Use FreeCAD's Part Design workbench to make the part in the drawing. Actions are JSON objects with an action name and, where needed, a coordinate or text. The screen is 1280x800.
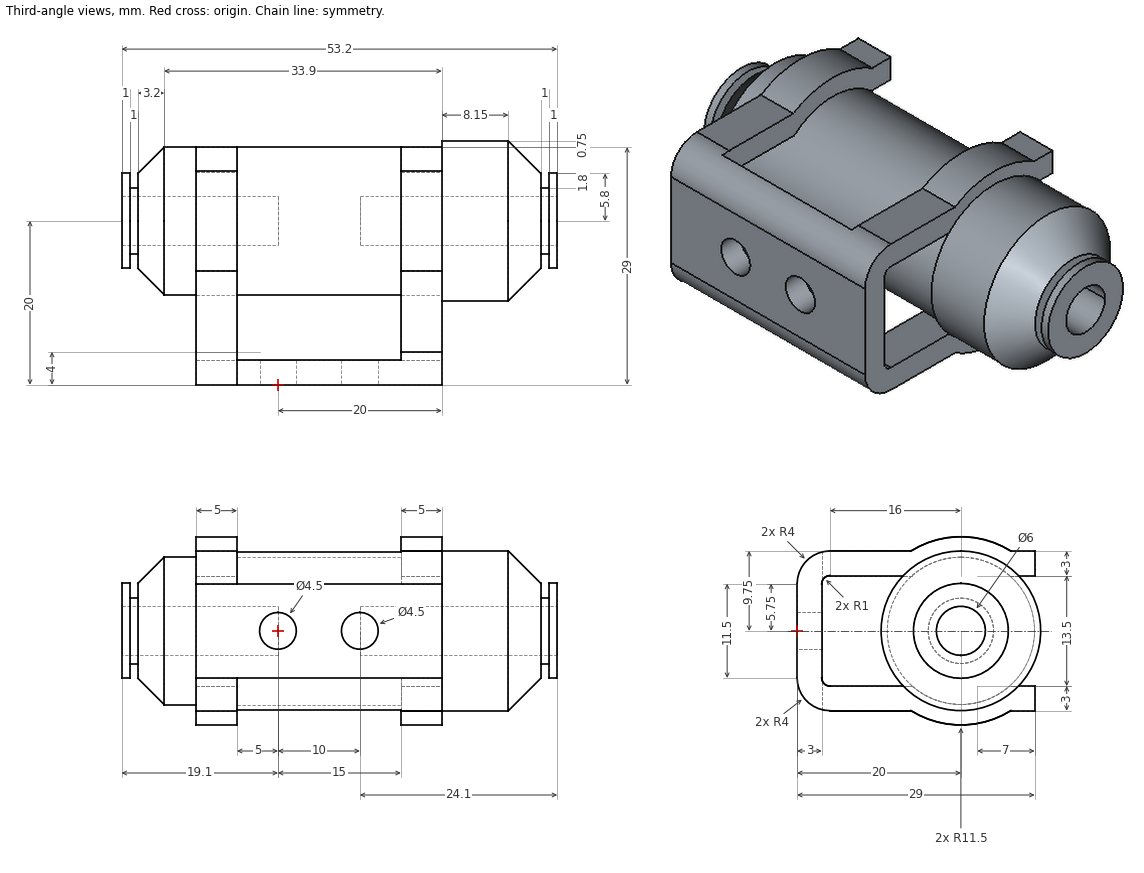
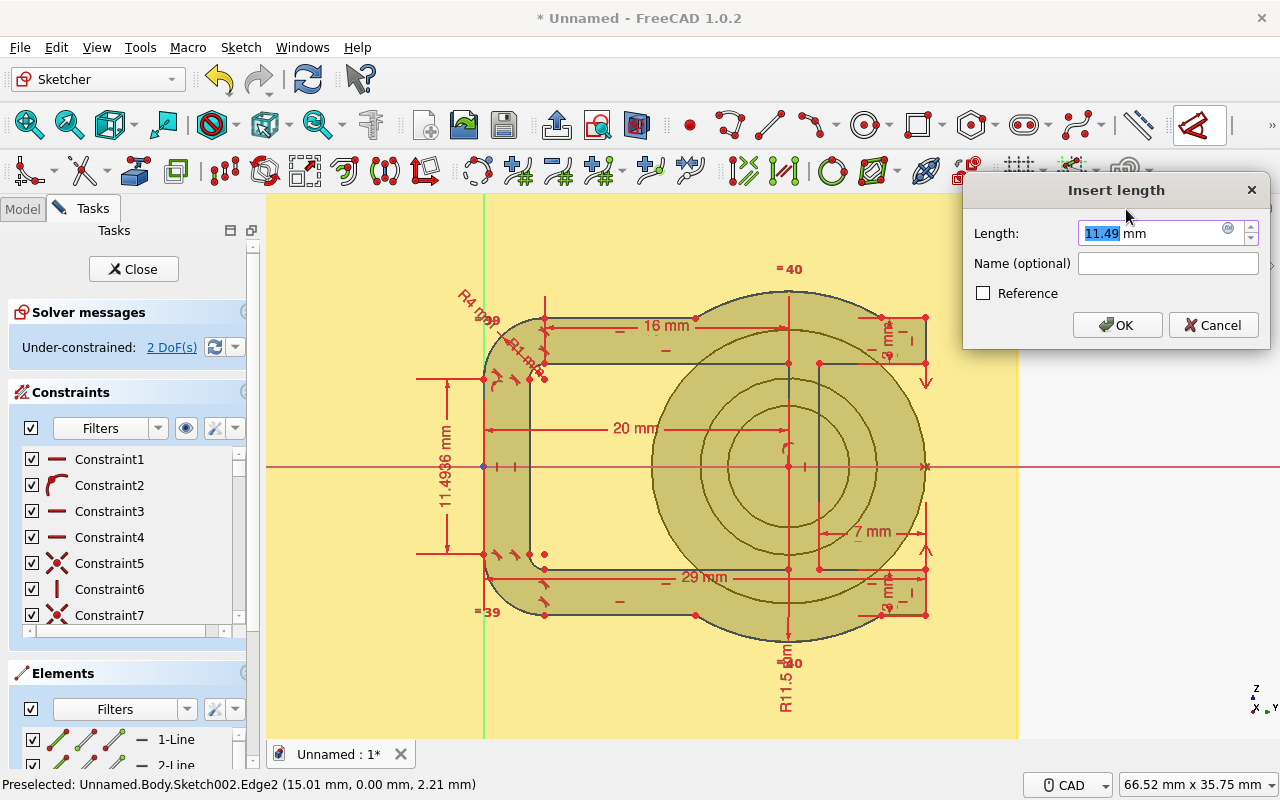
{"action": "type", "text": "11.5"}
{"action": "key", "text": "Return"}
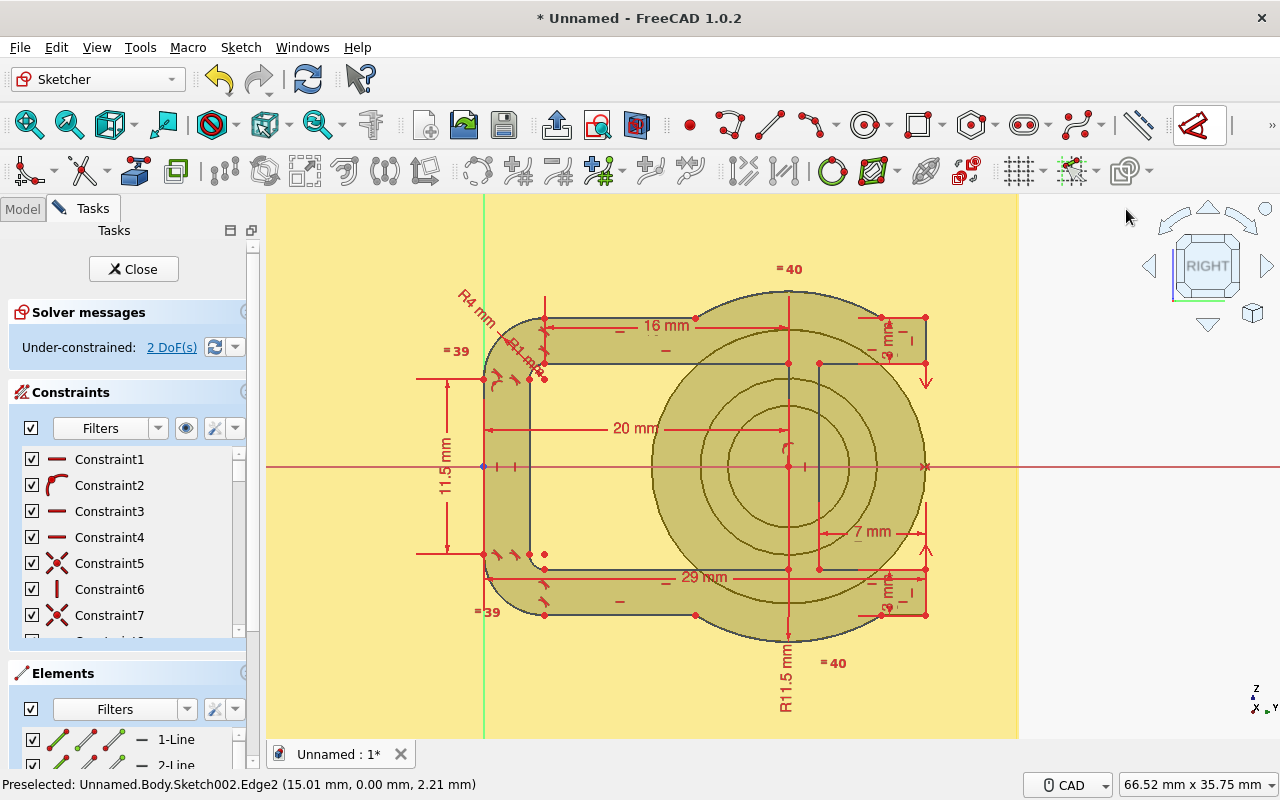
{"action": "left_click", "coordinate": [819, 508]}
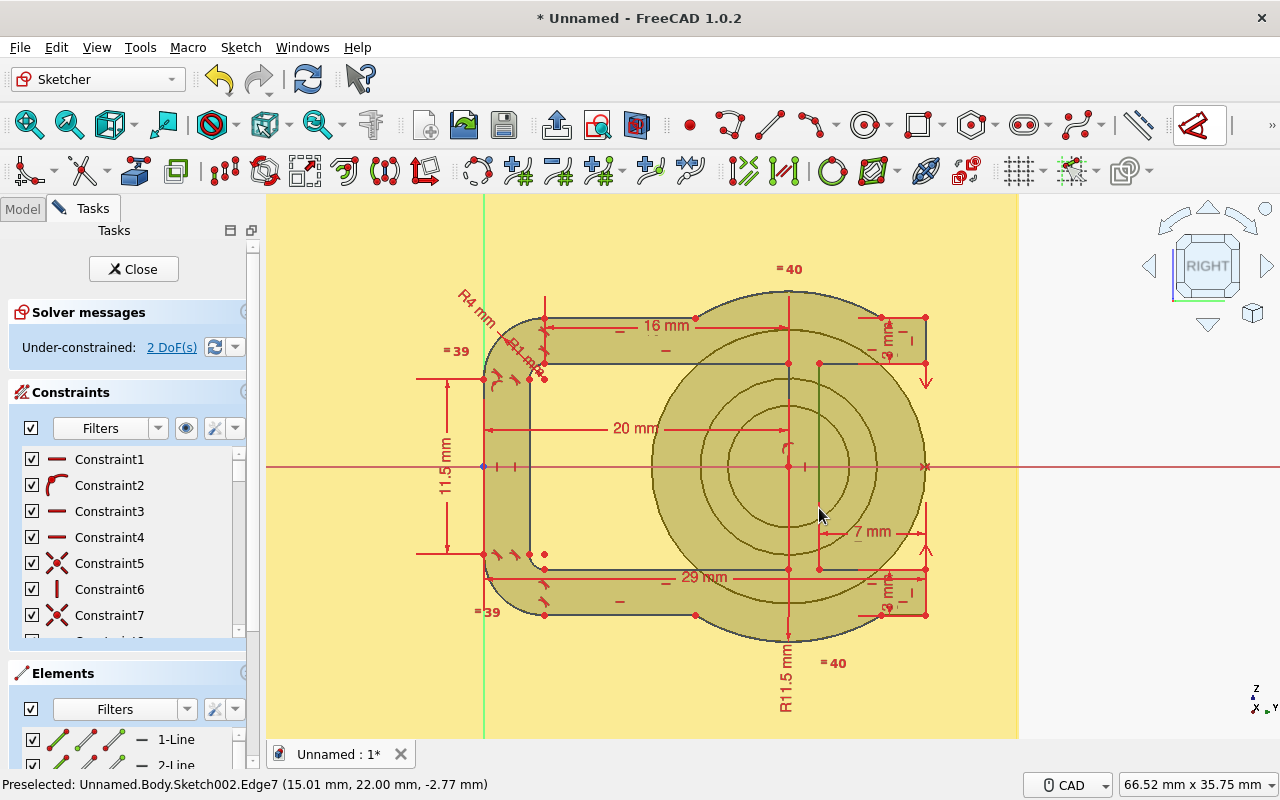
{"action": "left_click", "coordinate": [1220, 126]}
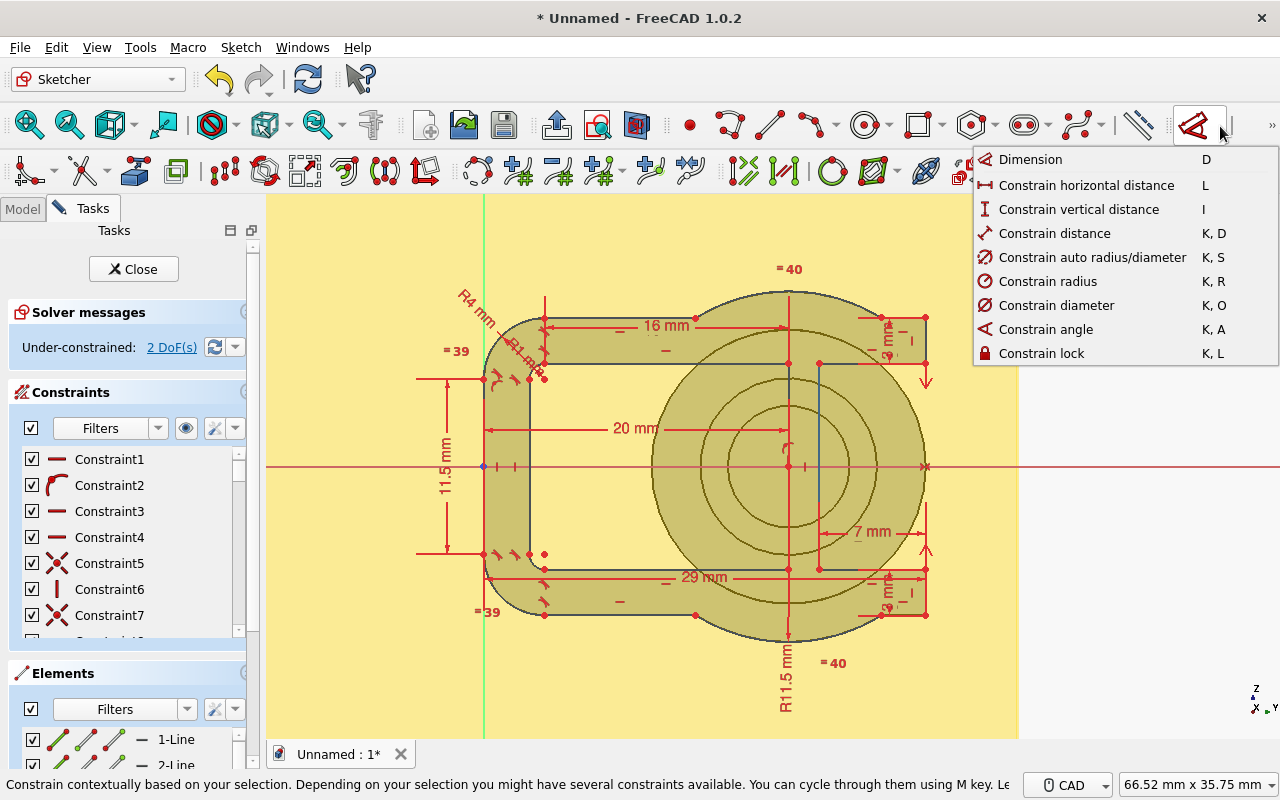
{"action": "left_click", "coordinate": [1126, 209]}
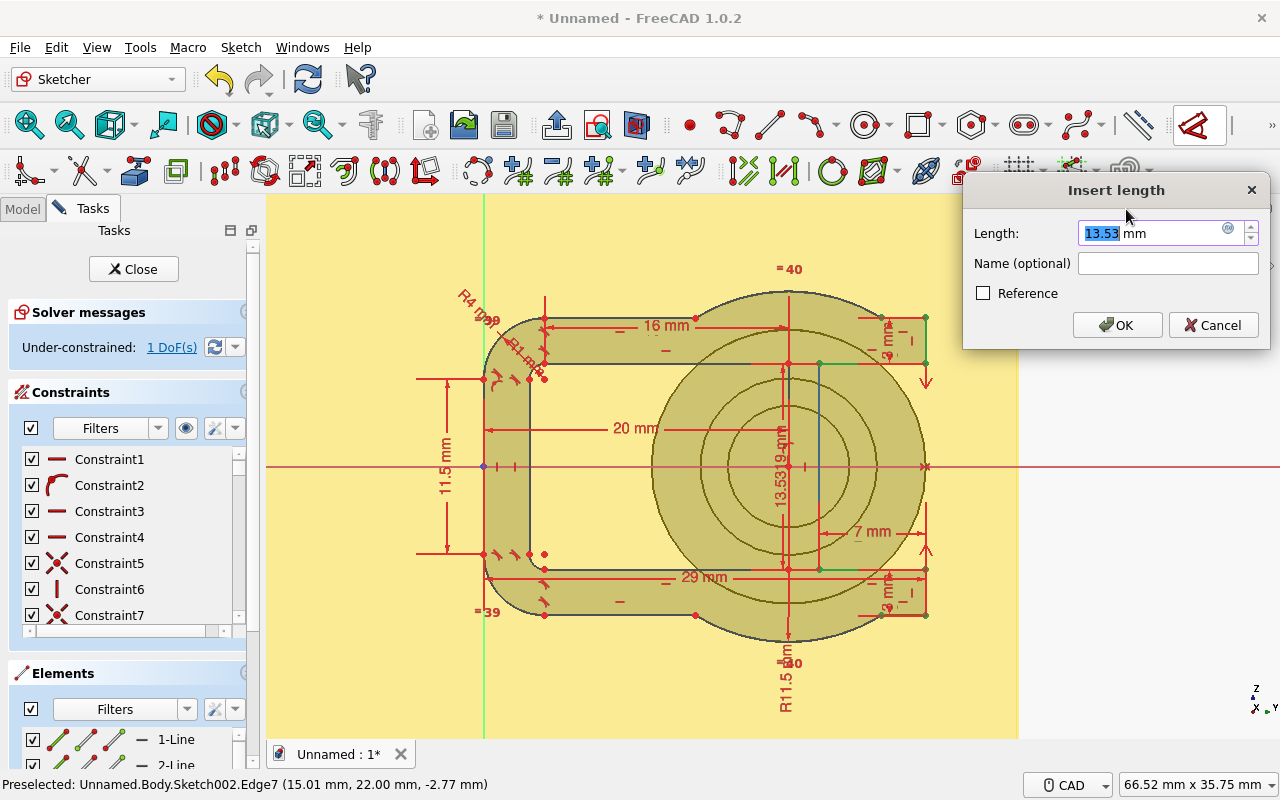
{"action": "type", "text": "13.5"}
{"action": "key", "text": "Return"}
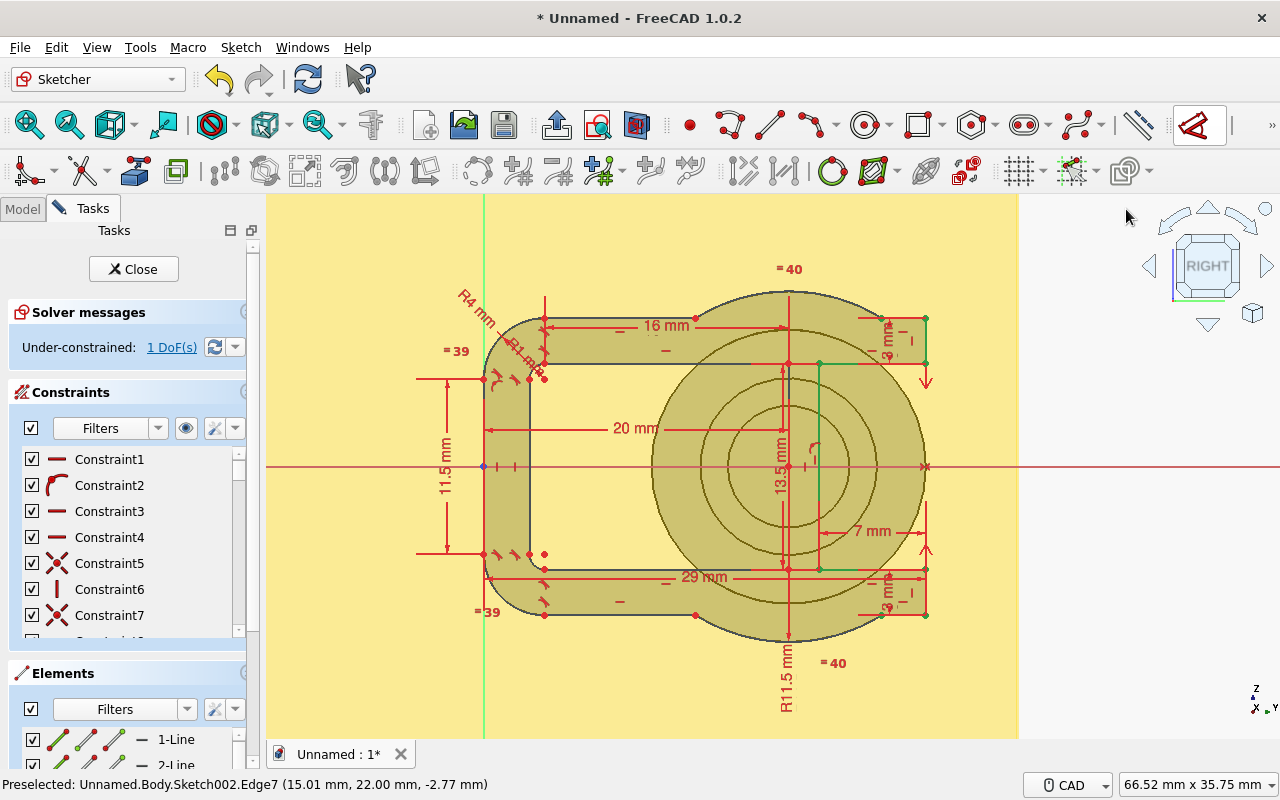
{"action": "left_click", "coordinate": [696, 318]}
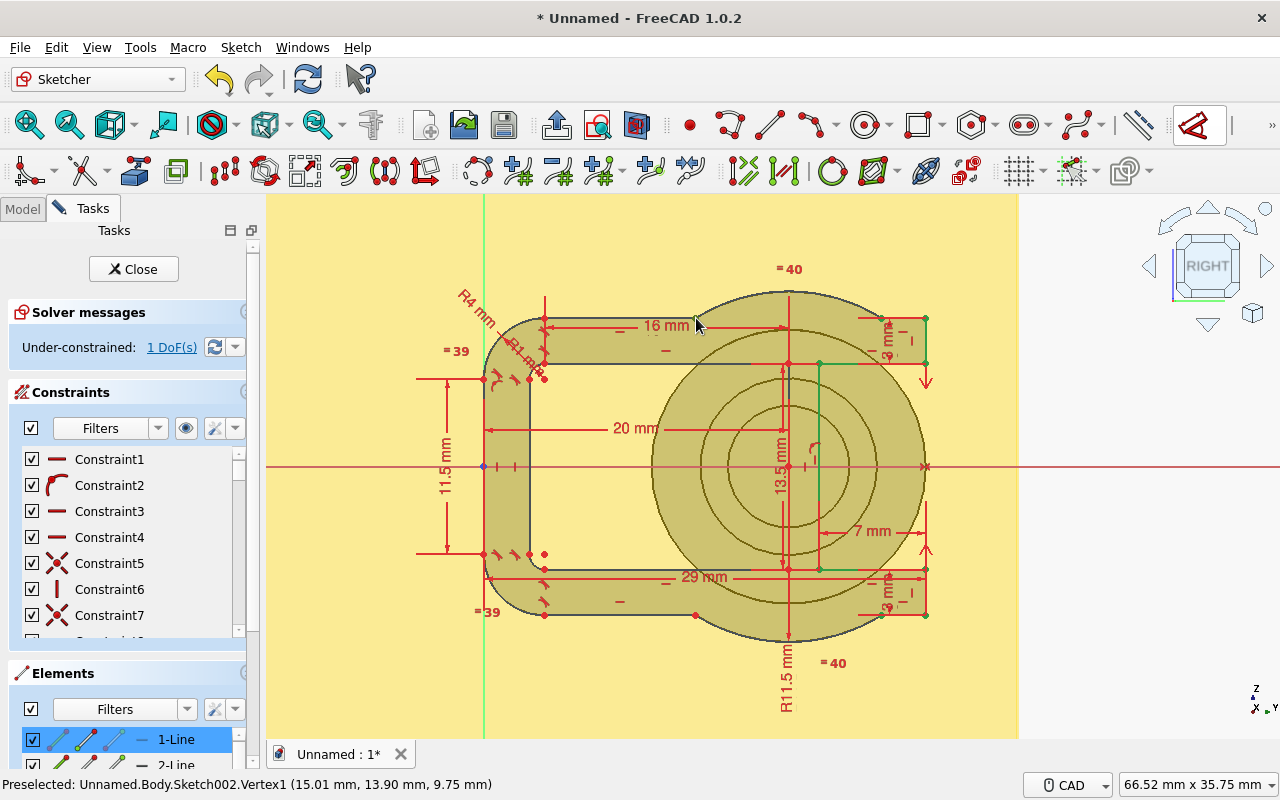
{"action": "left_click", "coordinate": [1220, 126]}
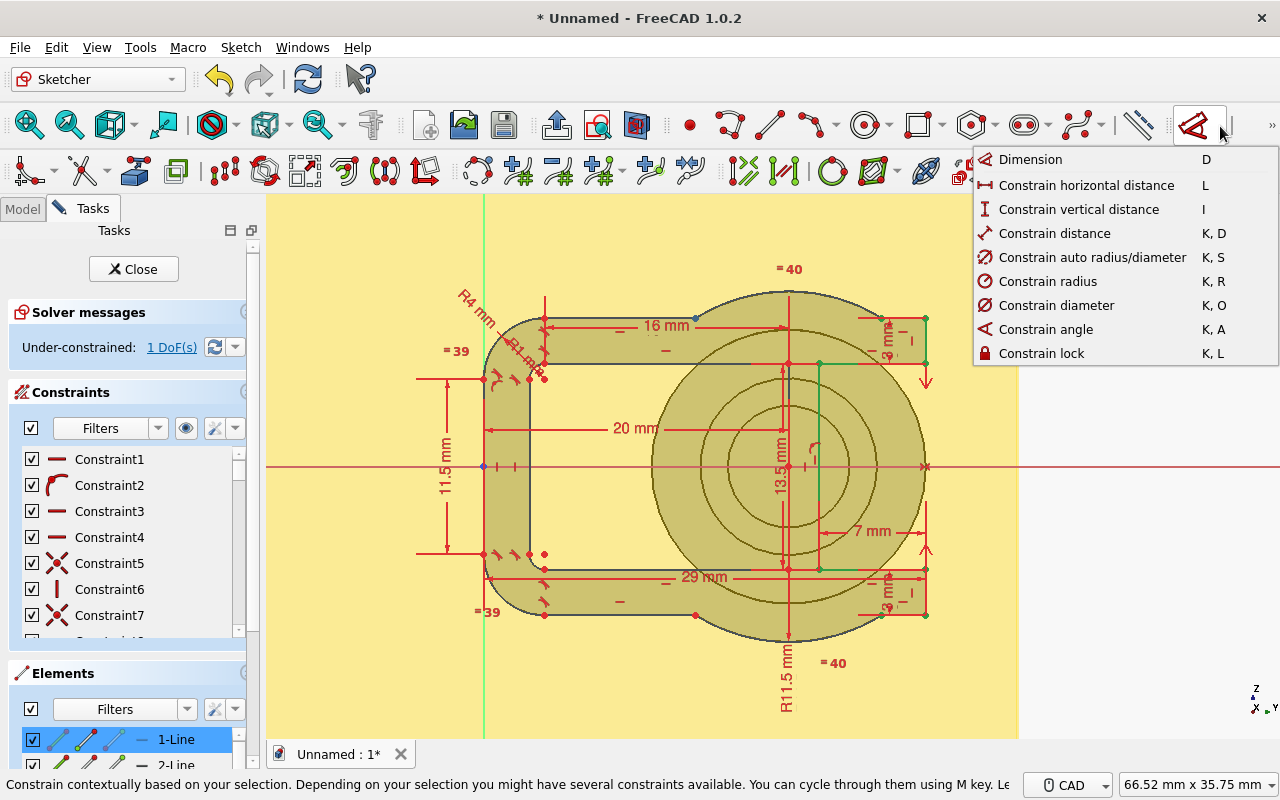
{"action": "left_click", "coordinate": [1126, 209]}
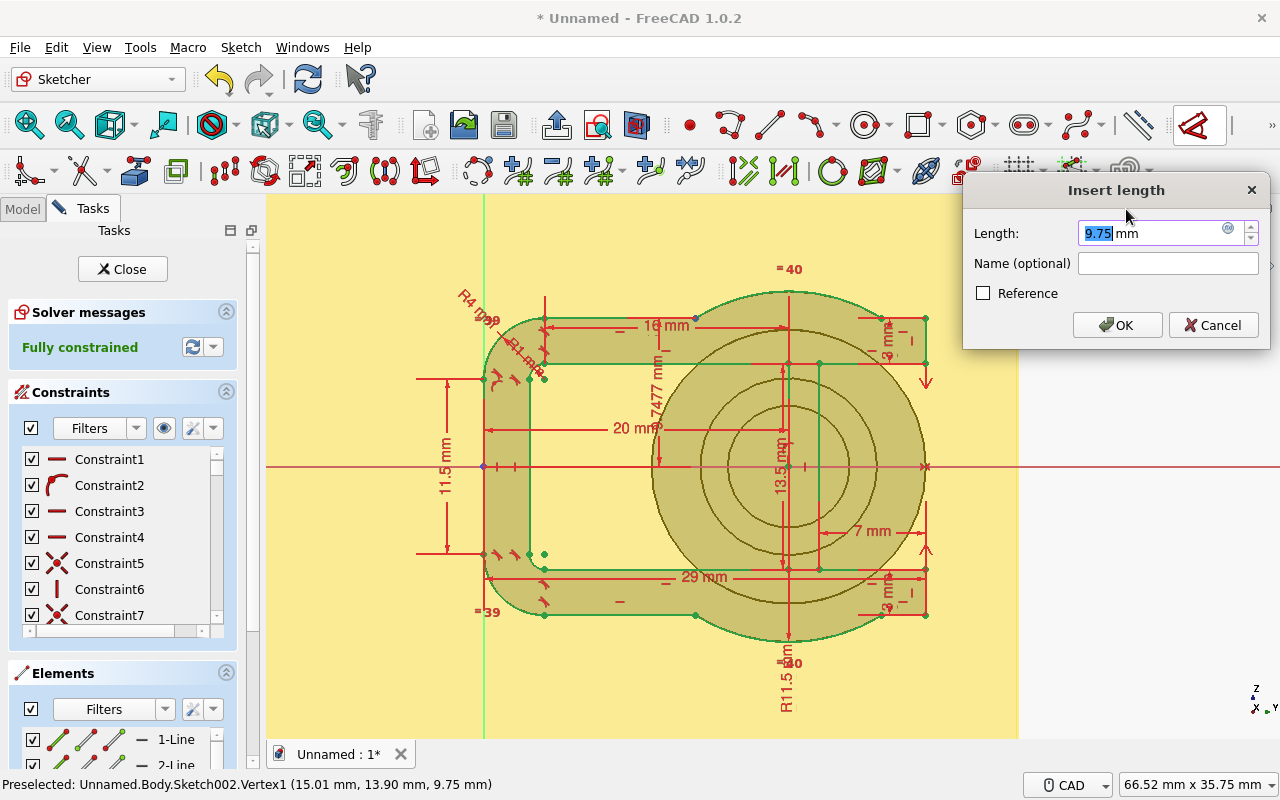
{"action": "type", "text": "9.75"}
{"action": "key", "text": "Return"}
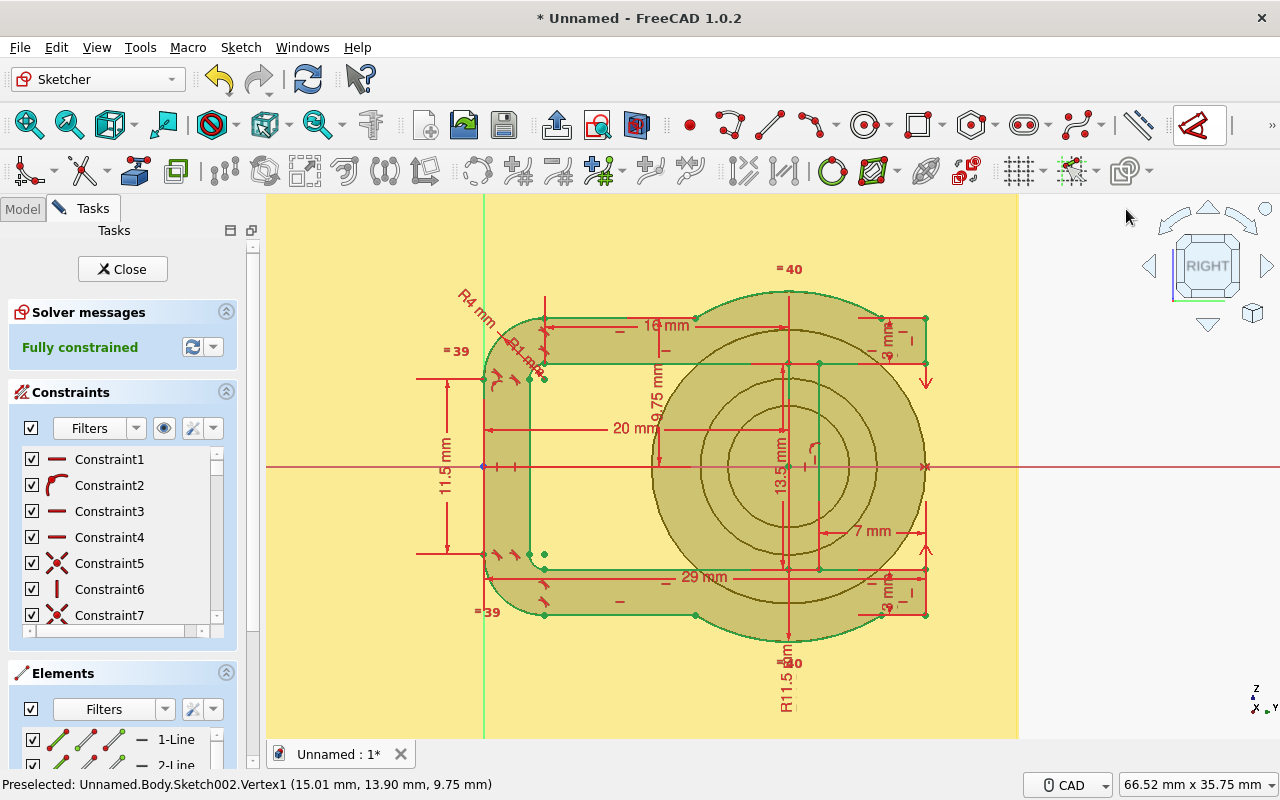
{"action": "left_click", "coordinate": [123, 269]}